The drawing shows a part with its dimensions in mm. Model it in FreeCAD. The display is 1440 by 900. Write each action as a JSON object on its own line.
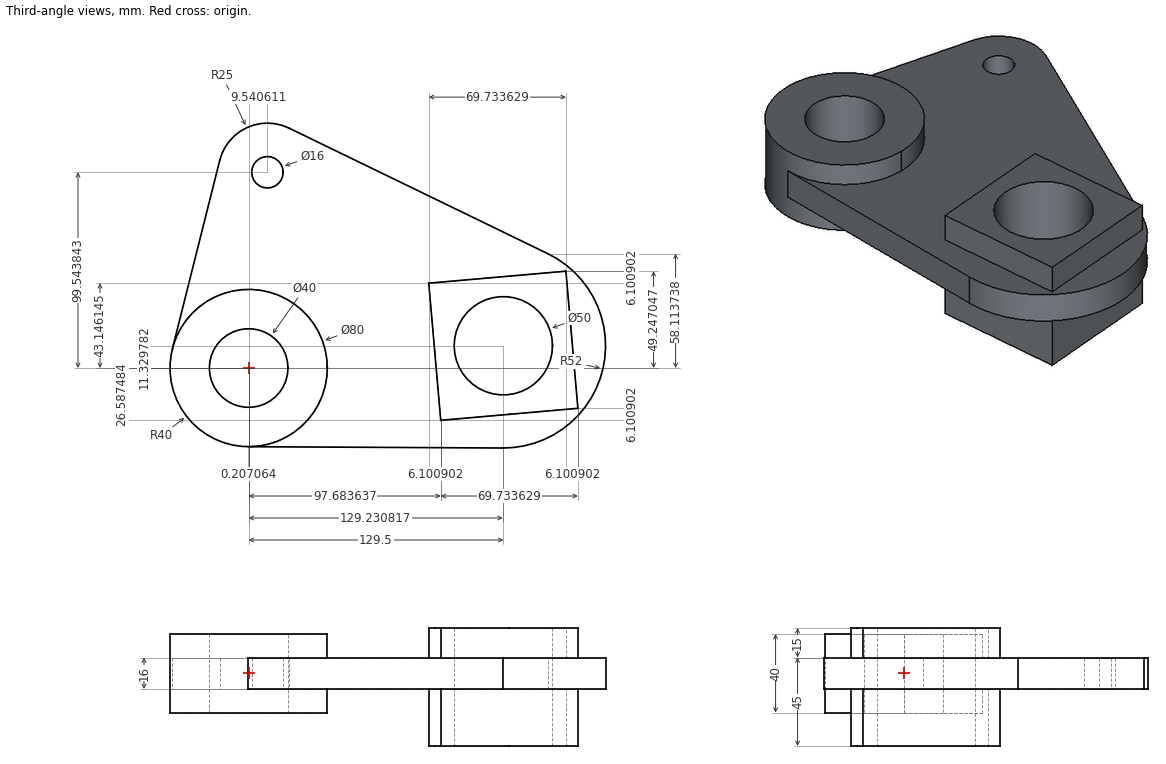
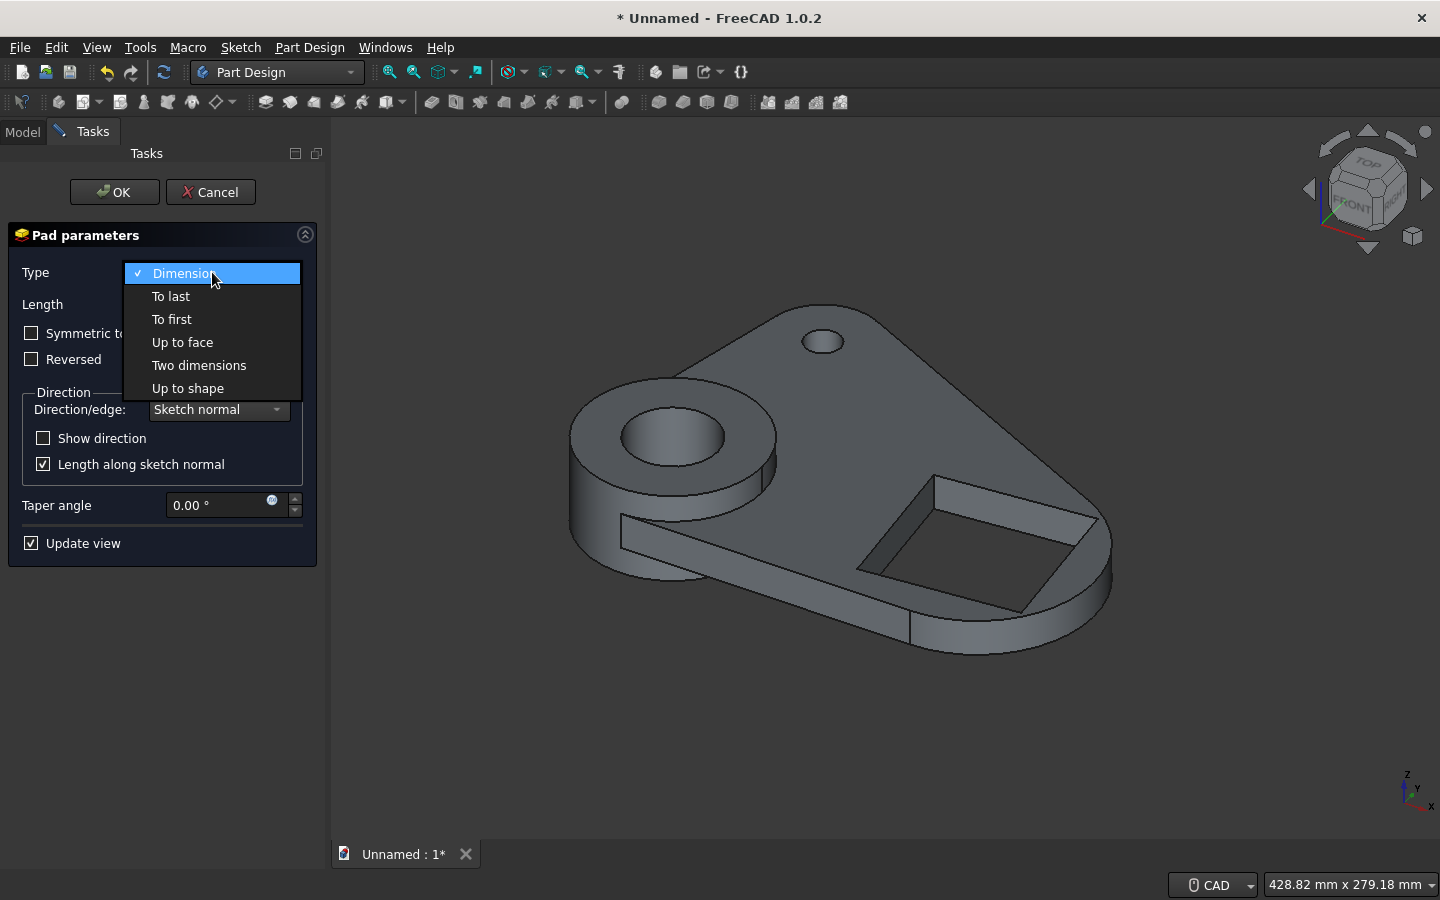
{"action": "left_click", "coordinate": [212, 366]}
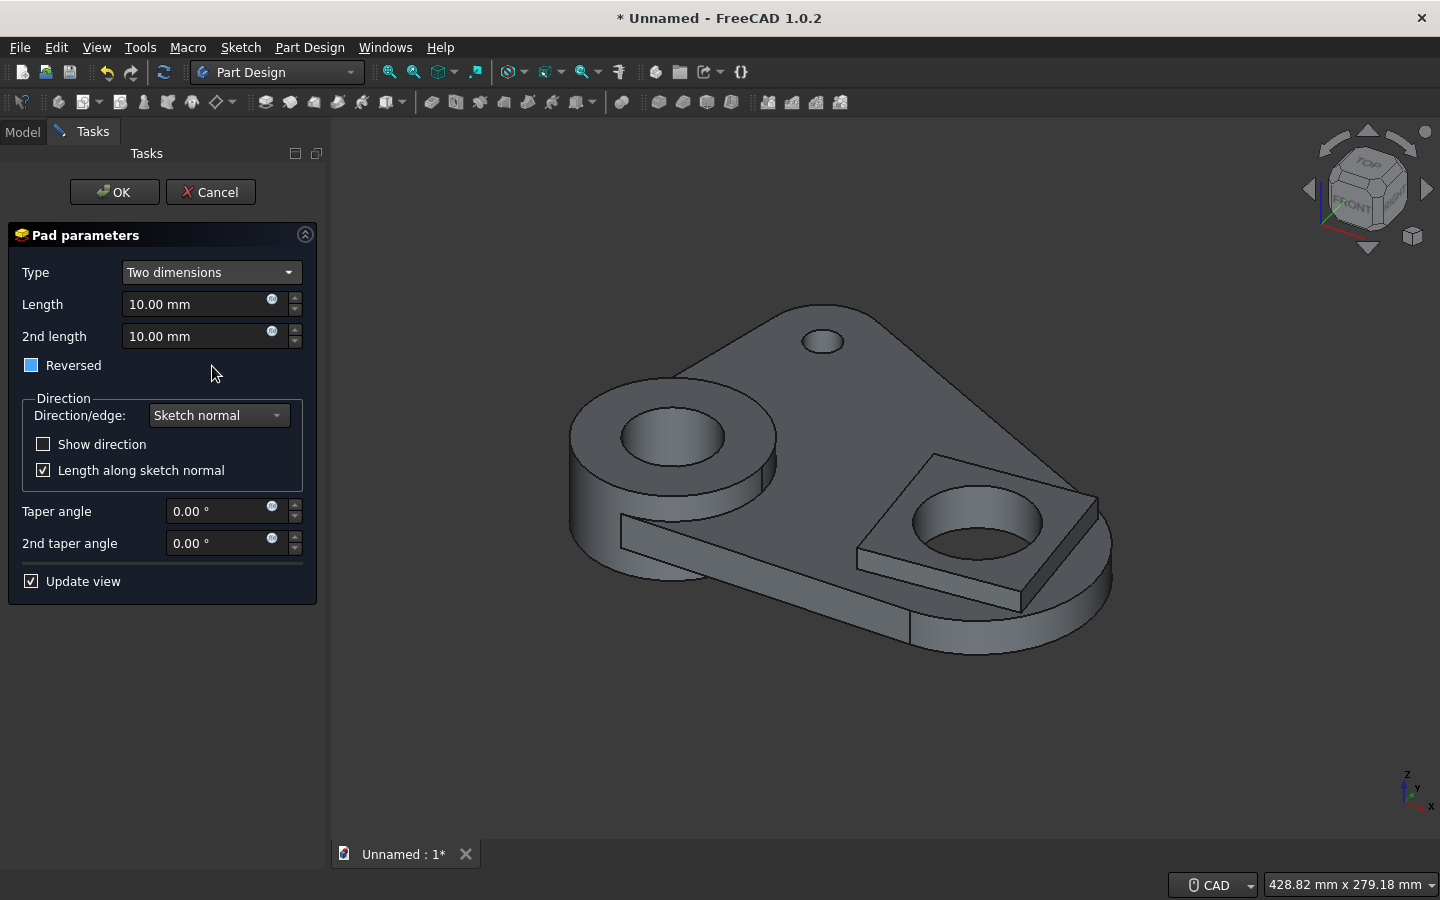
{"action": "triple_click", "coordinate": [204, 304]}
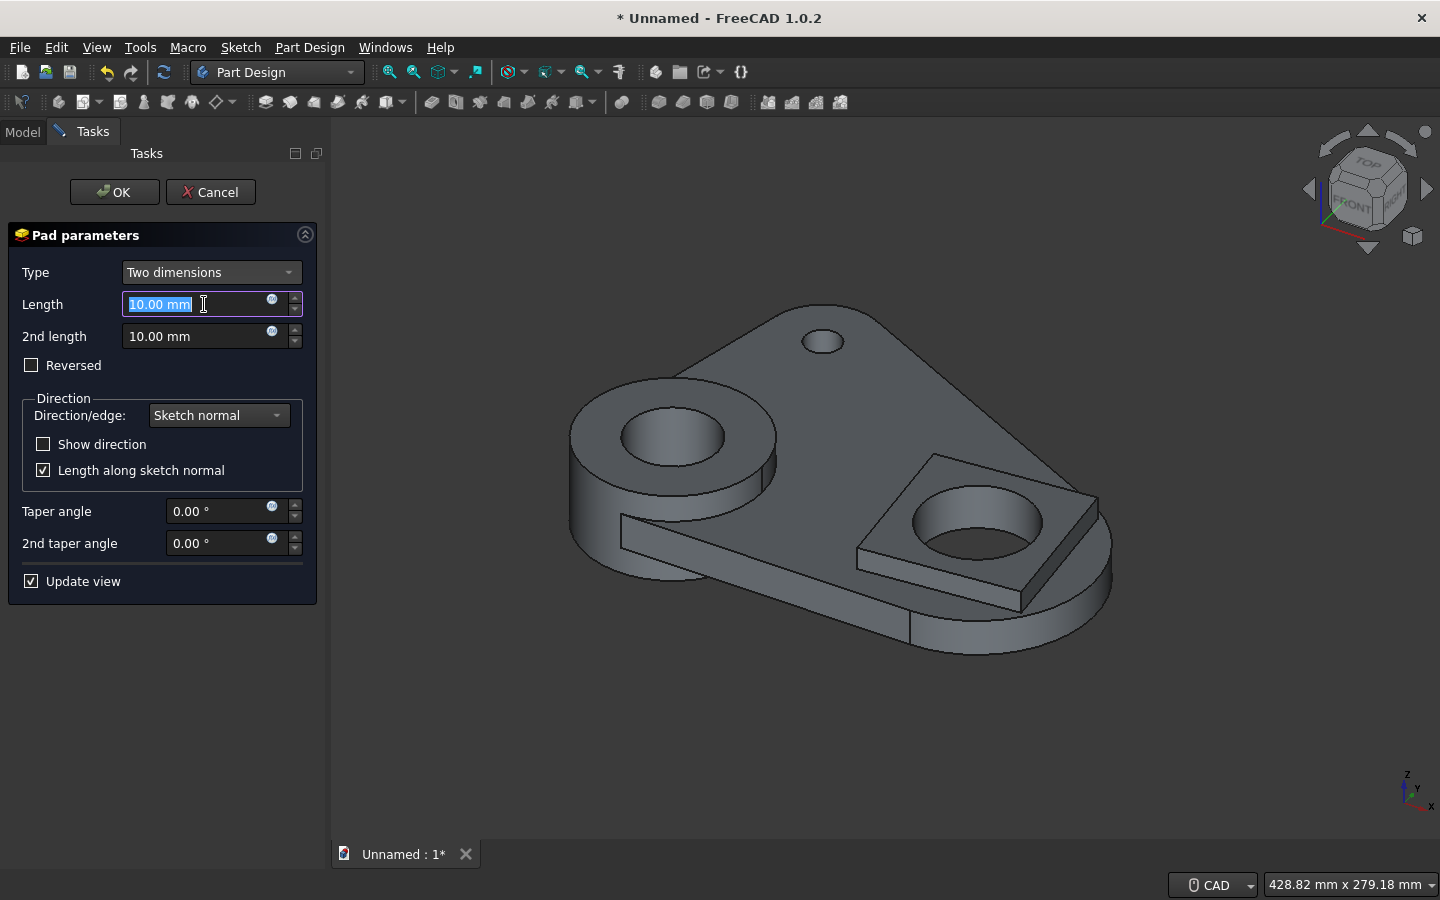
{"action": "type", "text": "15"}
{"action": "key", "text": "Tab"}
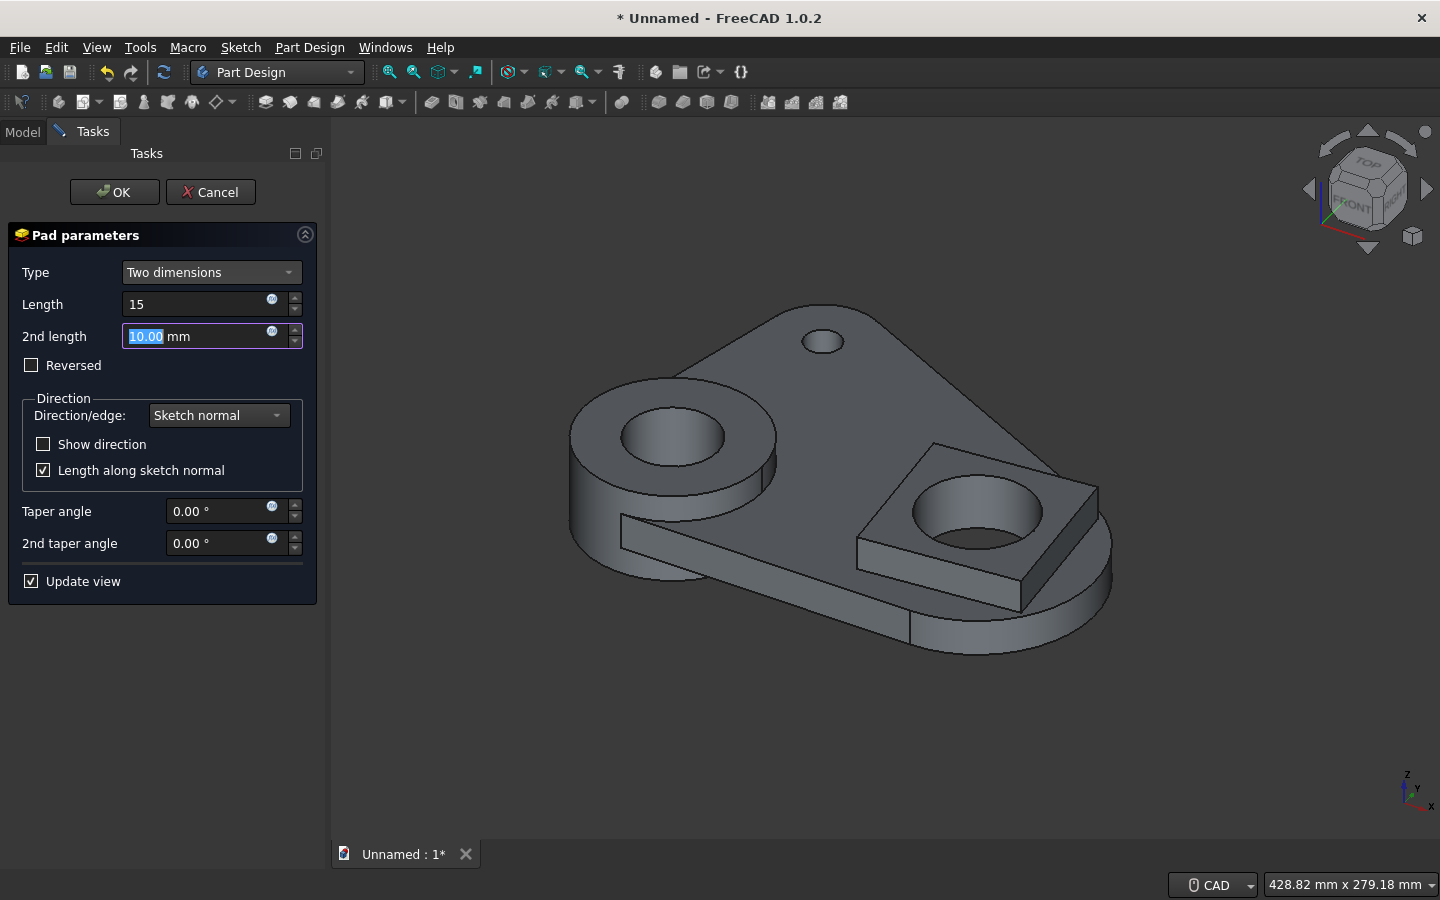
{"action": "type", "text": "45"}
{"action": "key", "text": "Tab"}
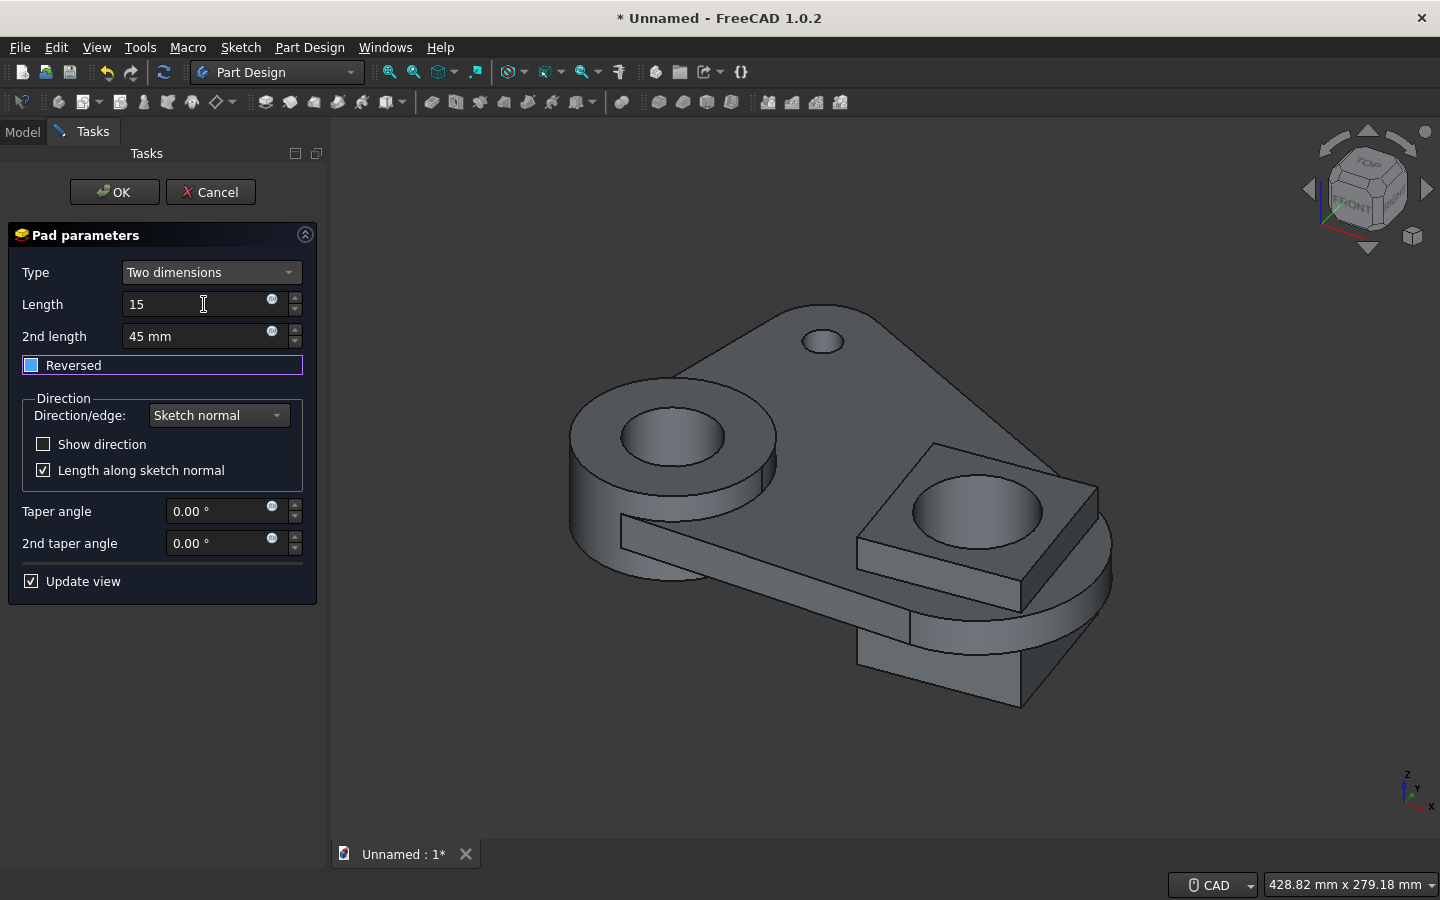
{"action": "left_click", "coordinate": [115, 192]}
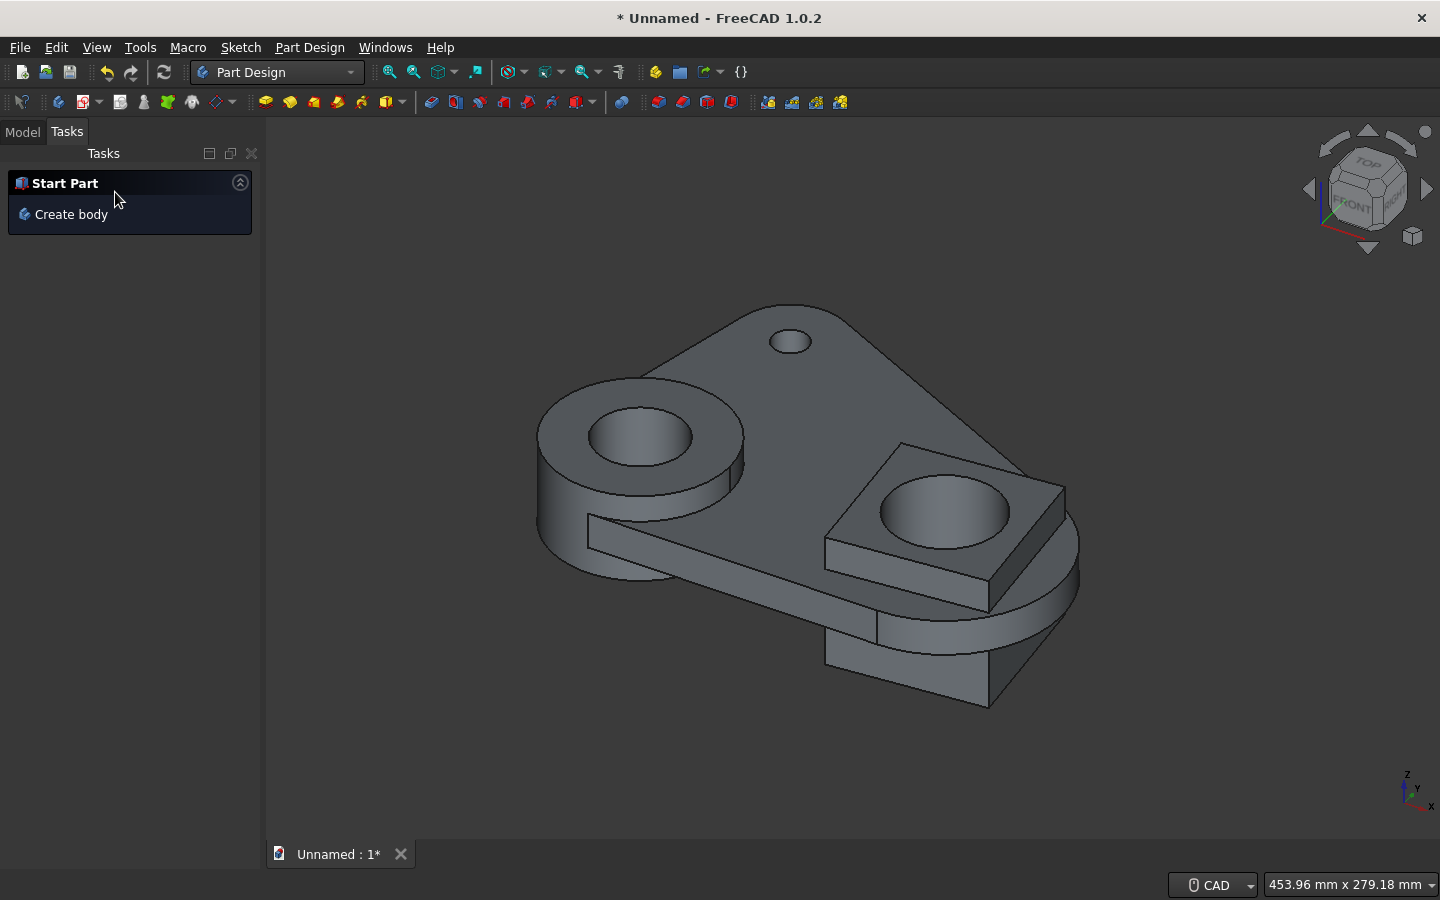
{"action": "key", "text": "0"}